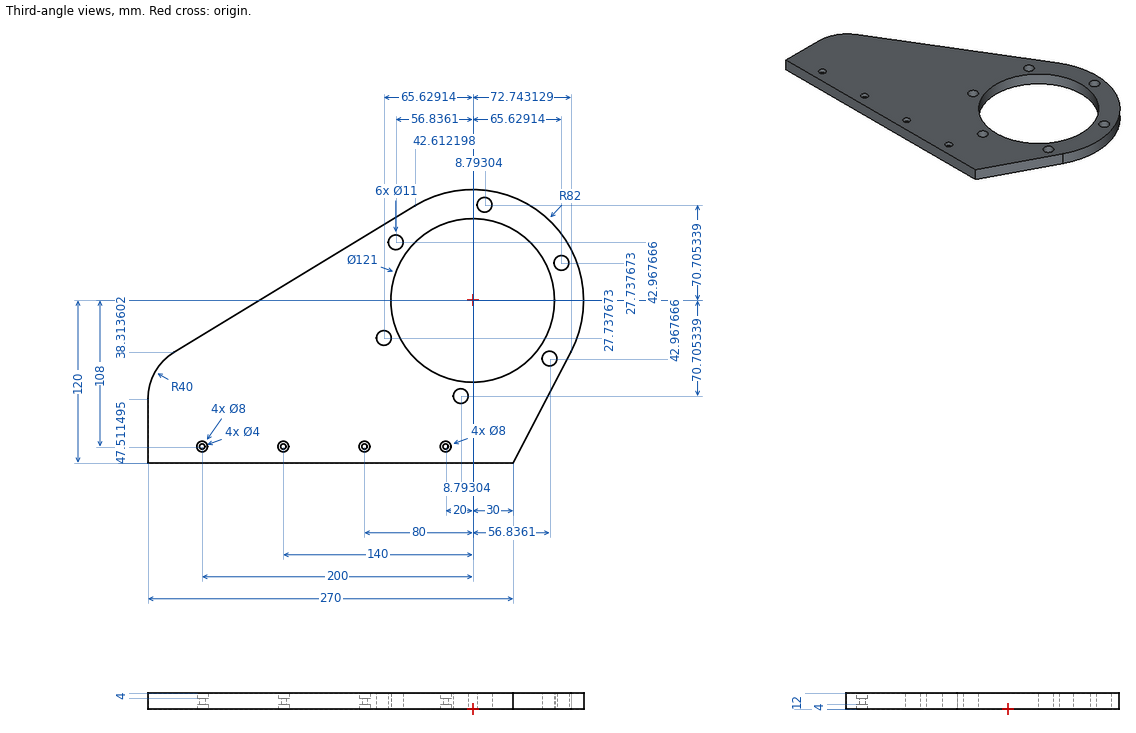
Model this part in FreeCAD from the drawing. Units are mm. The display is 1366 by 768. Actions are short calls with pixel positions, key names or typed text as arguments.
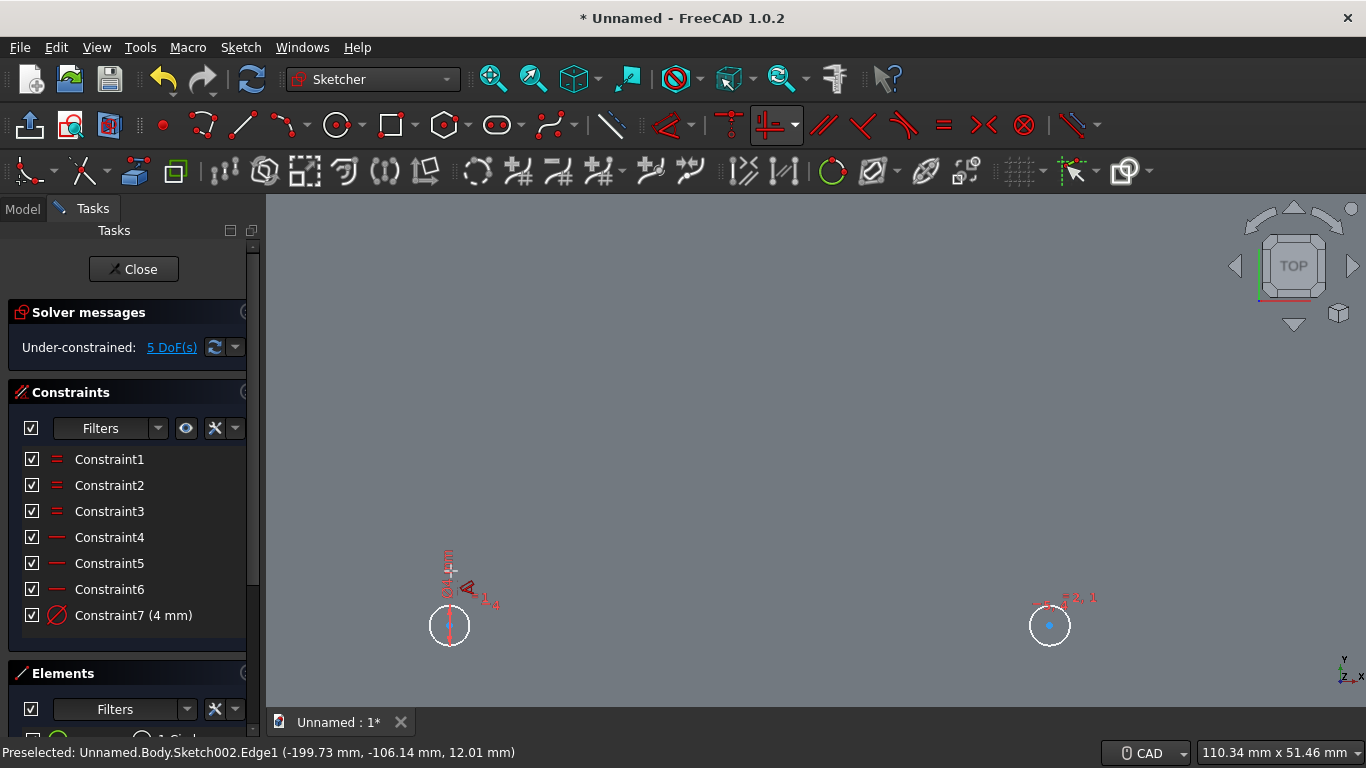
scroll(450, 604, down, 6)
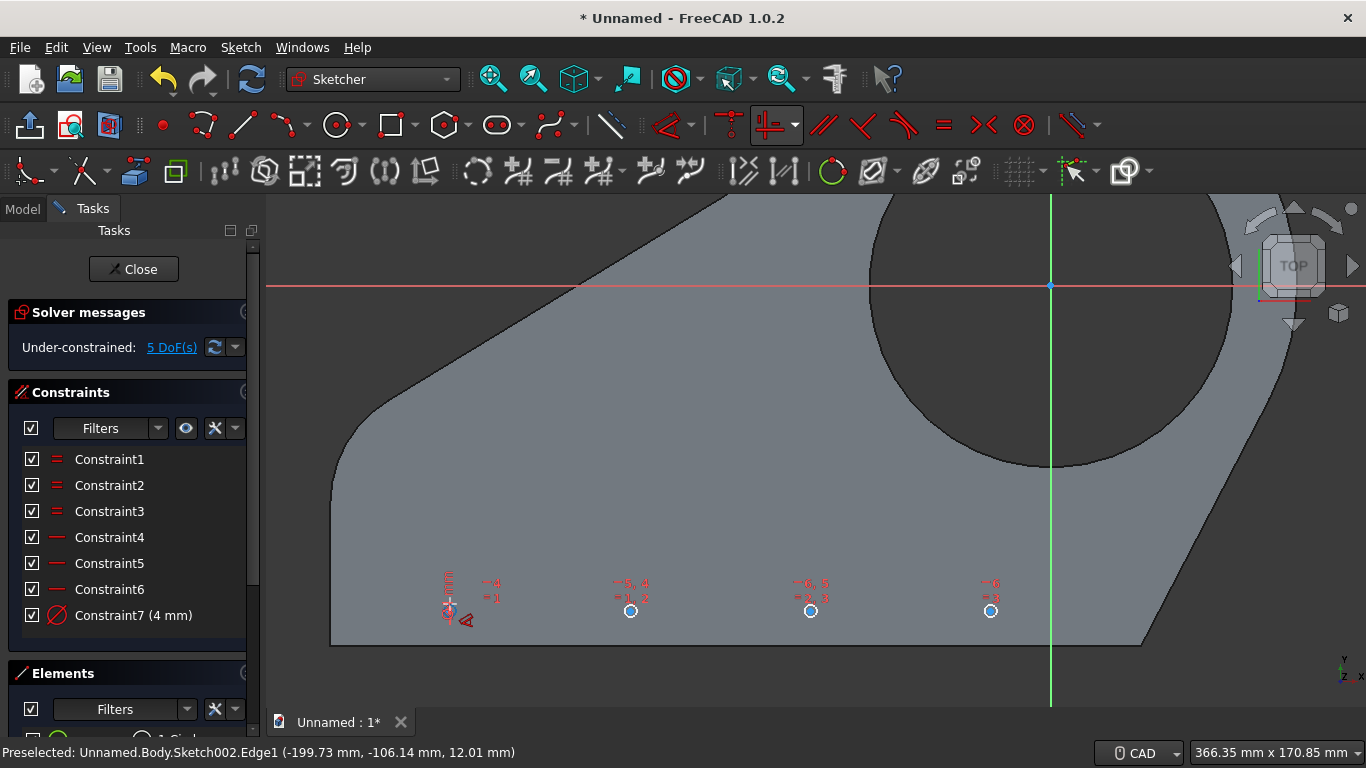
click(811, 611)
click(931, 252)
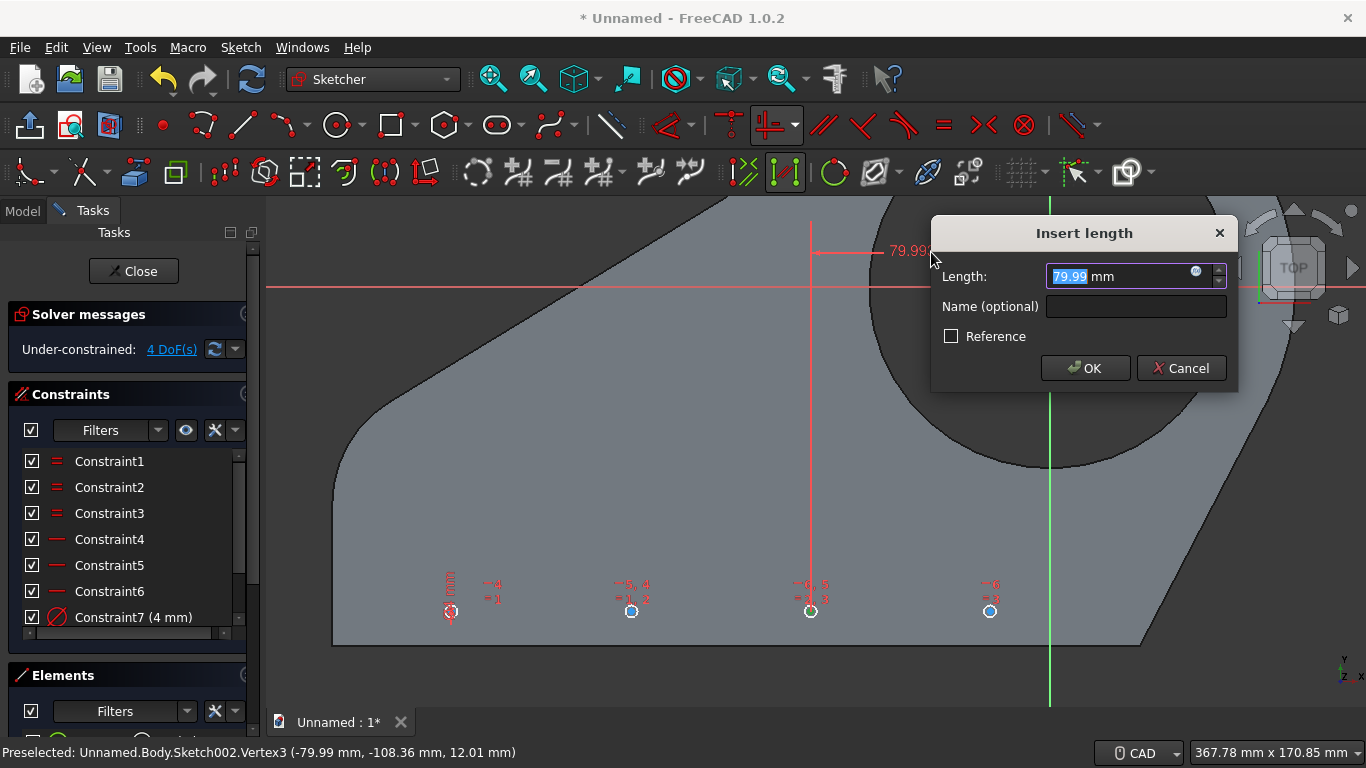
text(80)
key(Return)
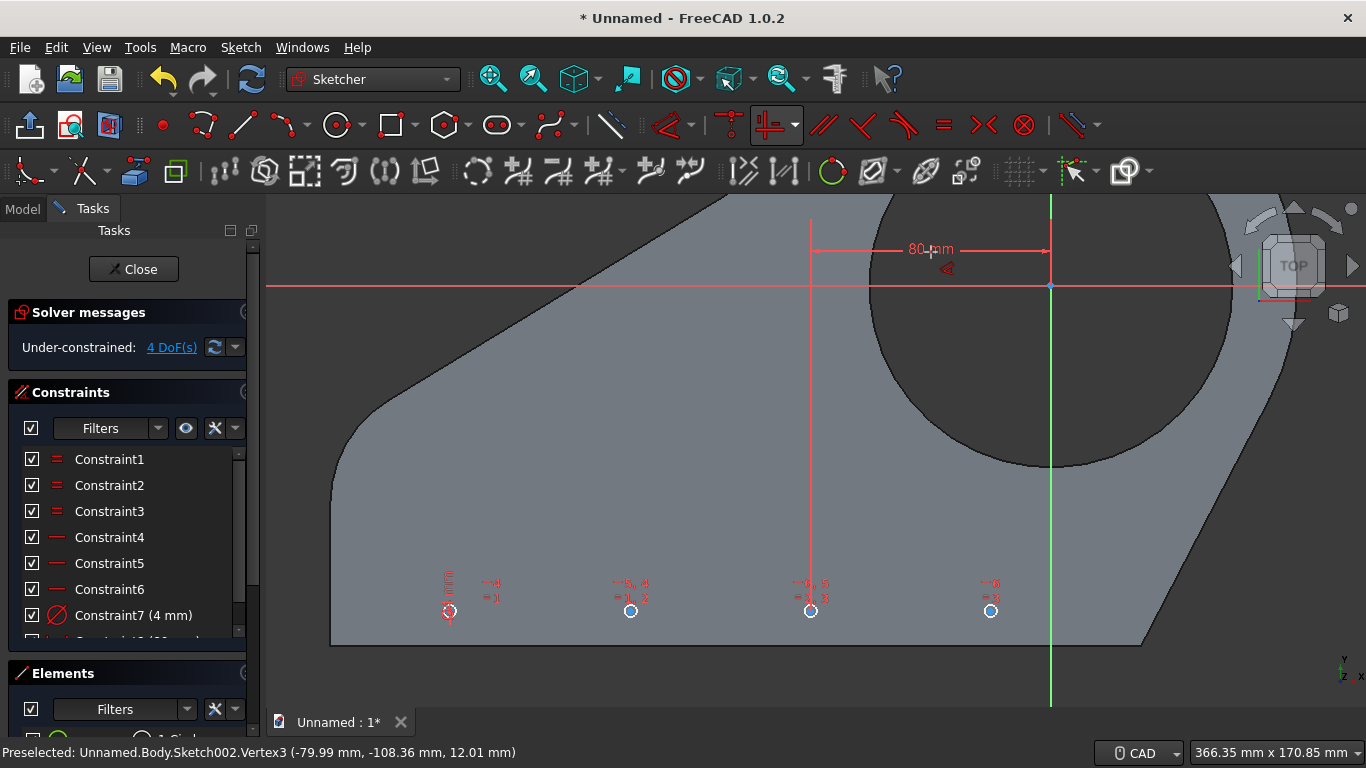
click(991, 611)
click(1021, 252)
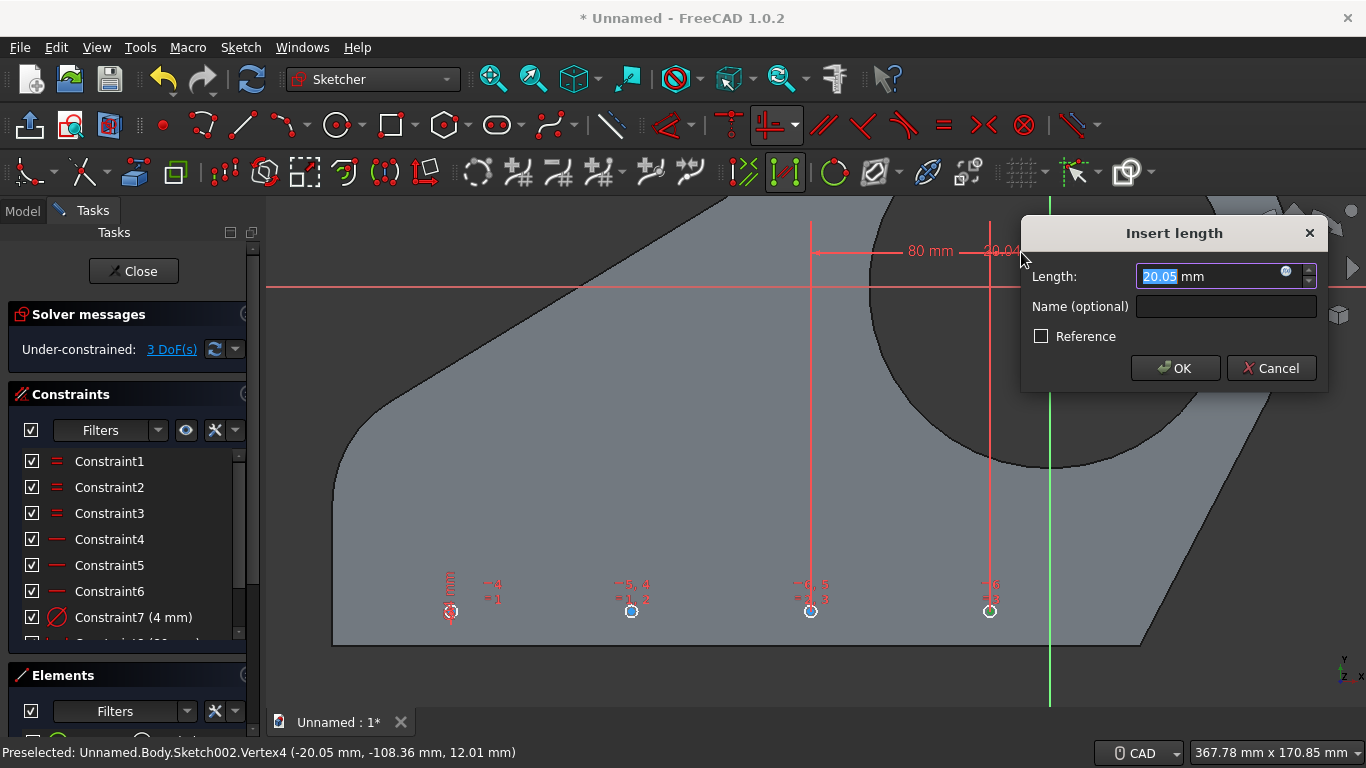
text(20)
key(Return)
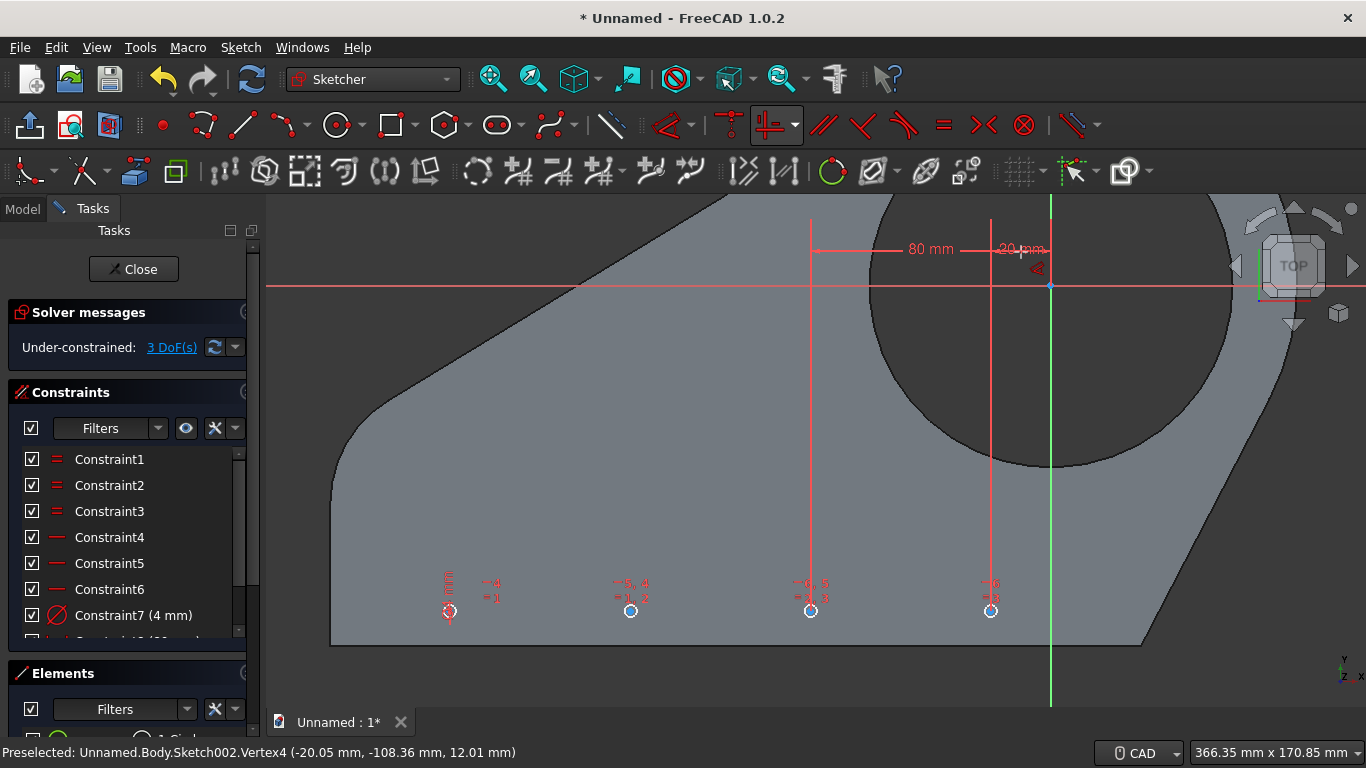
click(450, 611)
click(750, 252)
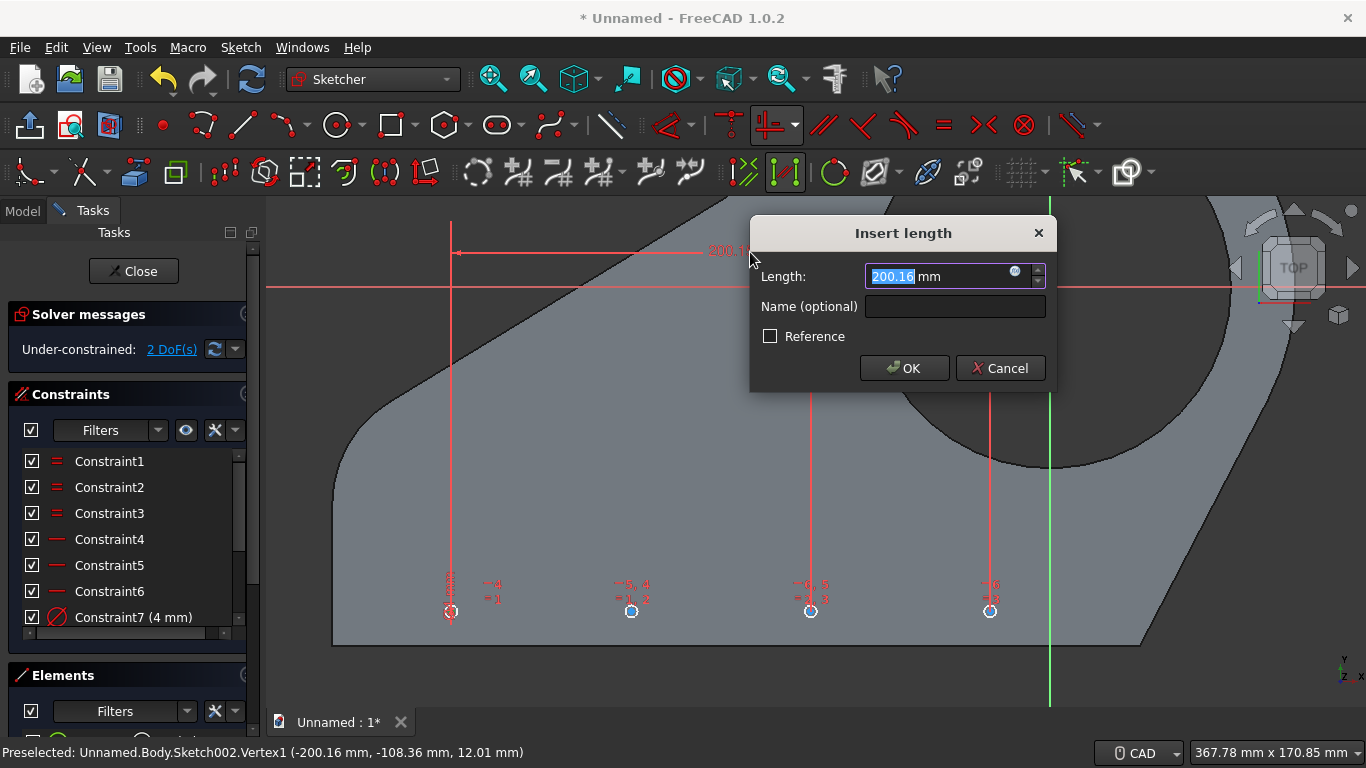
text(200)
key(Return)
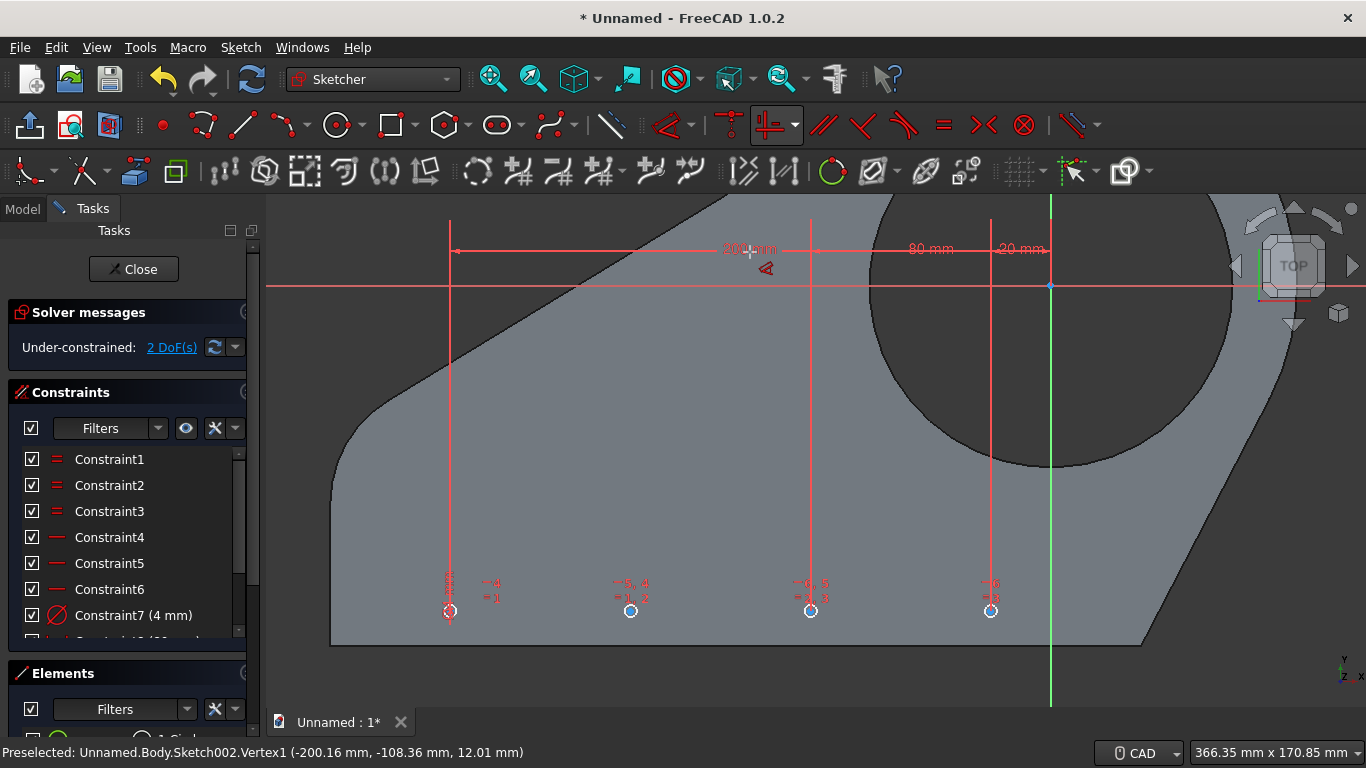
click(450, 611)
click(1085, 448)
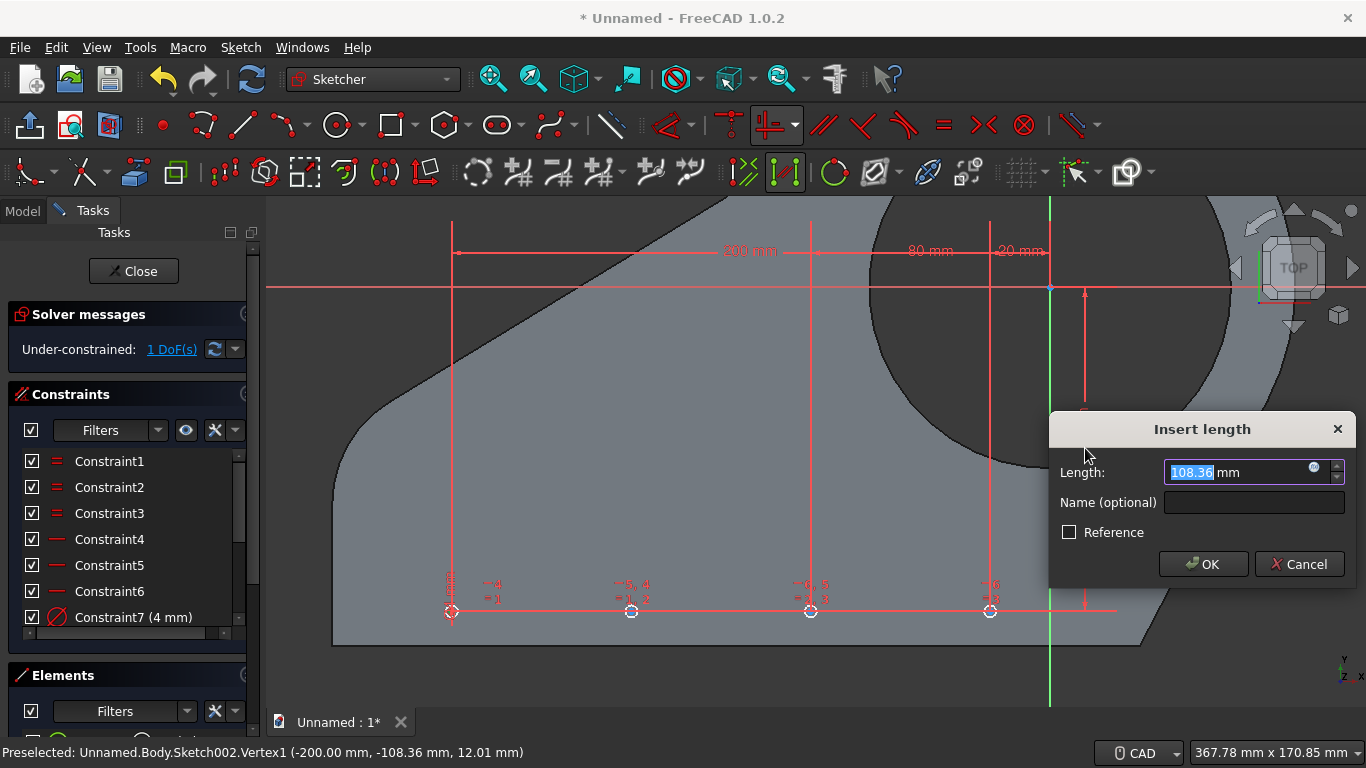
text(108)
key(Return)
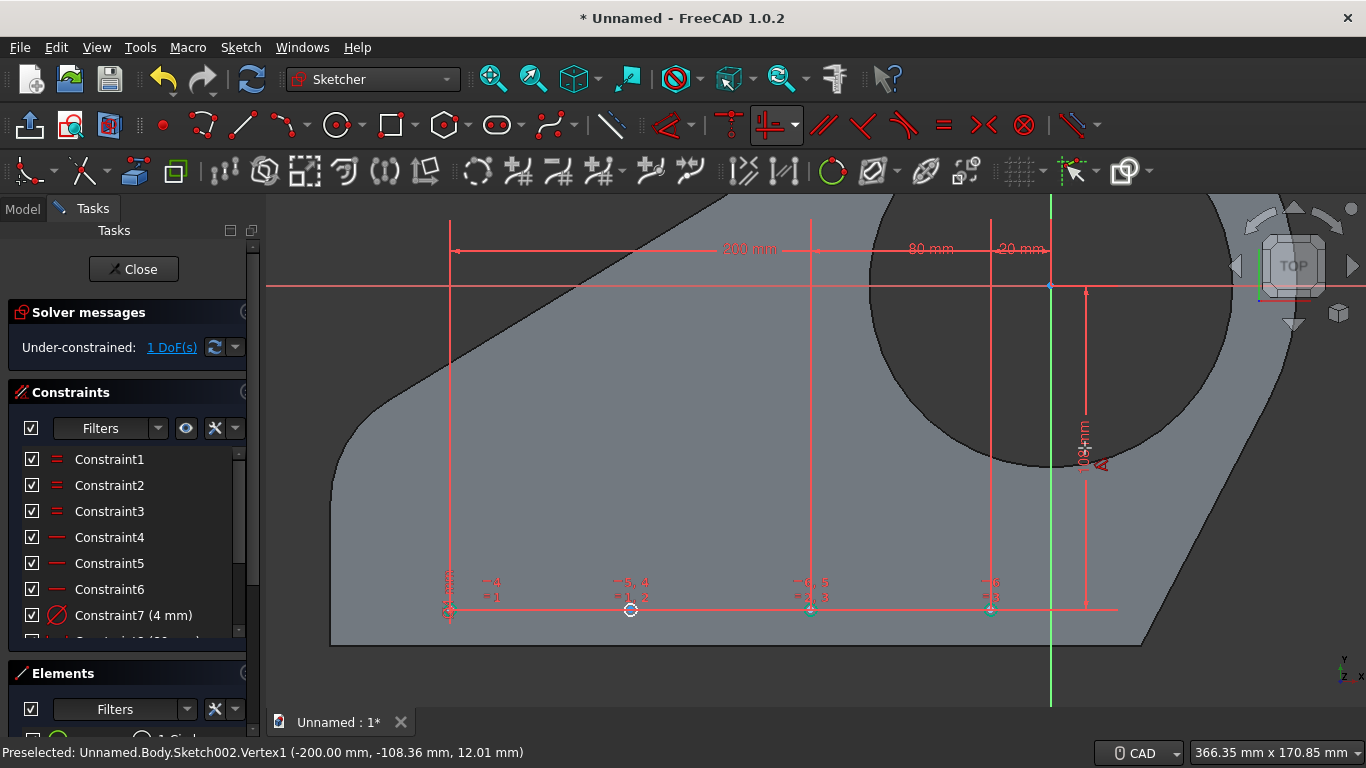
click(631, 610)
click(841, 252)